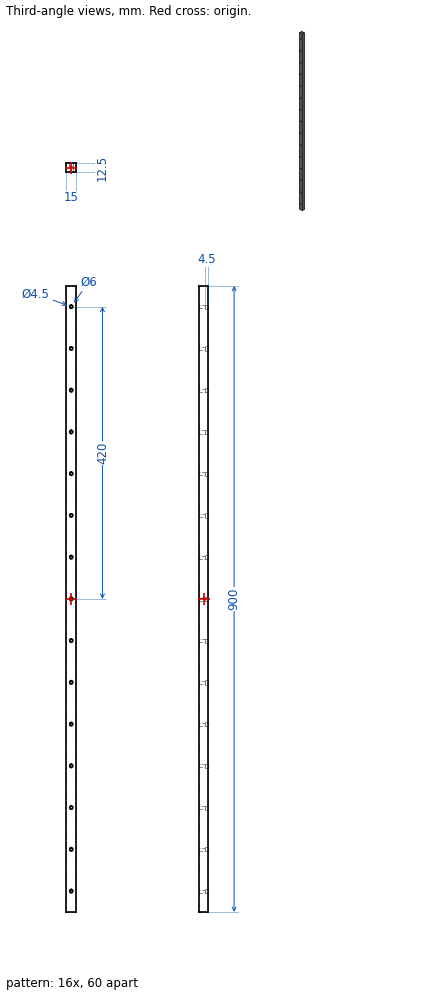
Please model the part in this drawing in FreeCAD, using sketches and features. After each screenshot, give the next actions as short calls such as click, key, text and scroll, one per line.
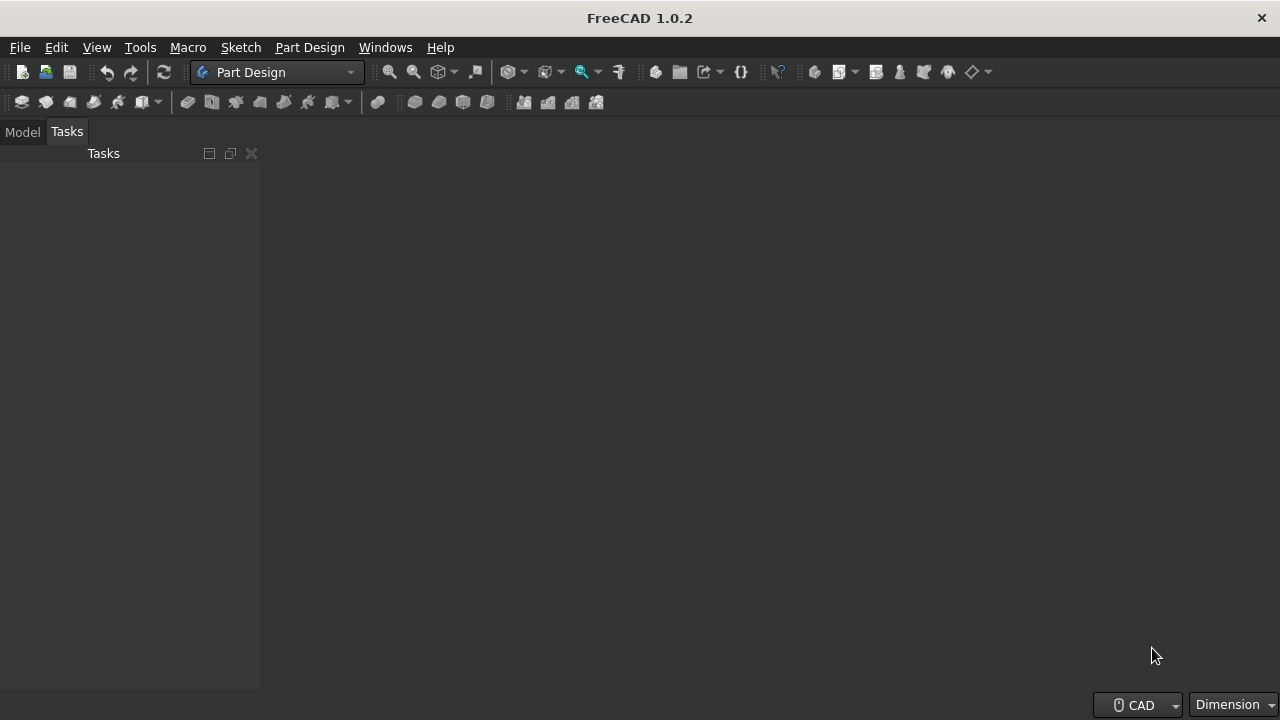
click(22, 72)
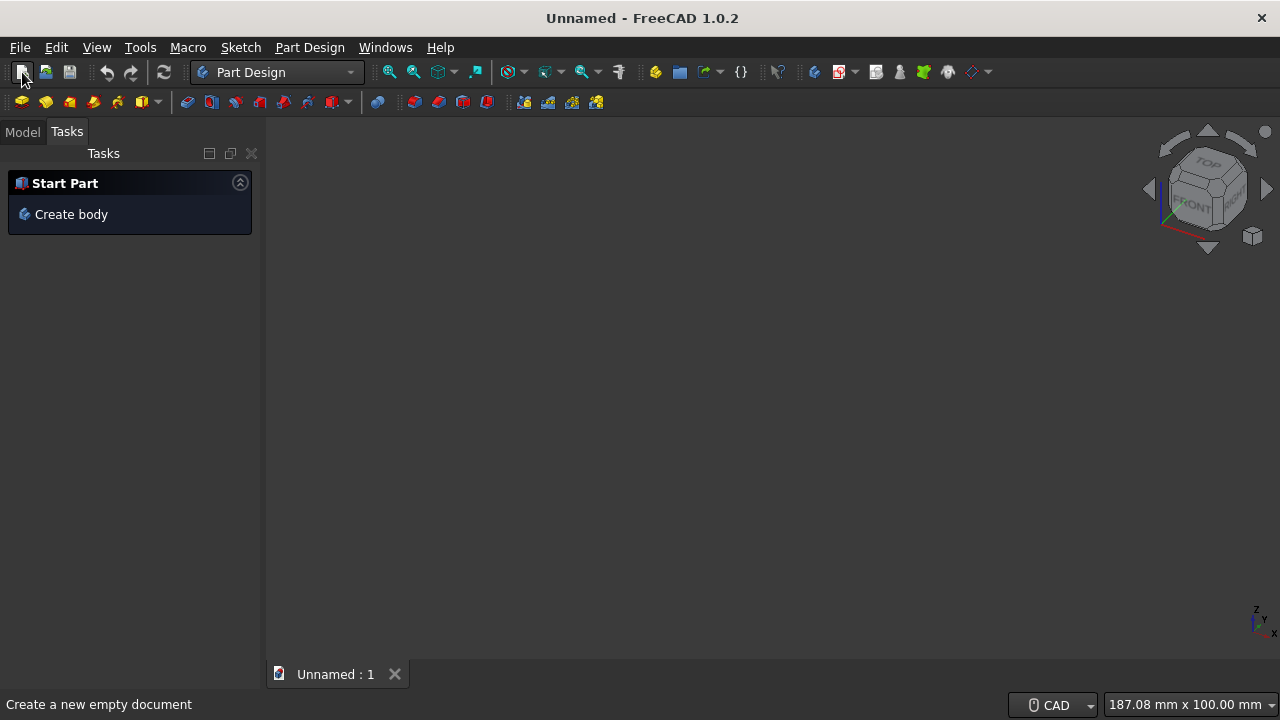
click(840, 72)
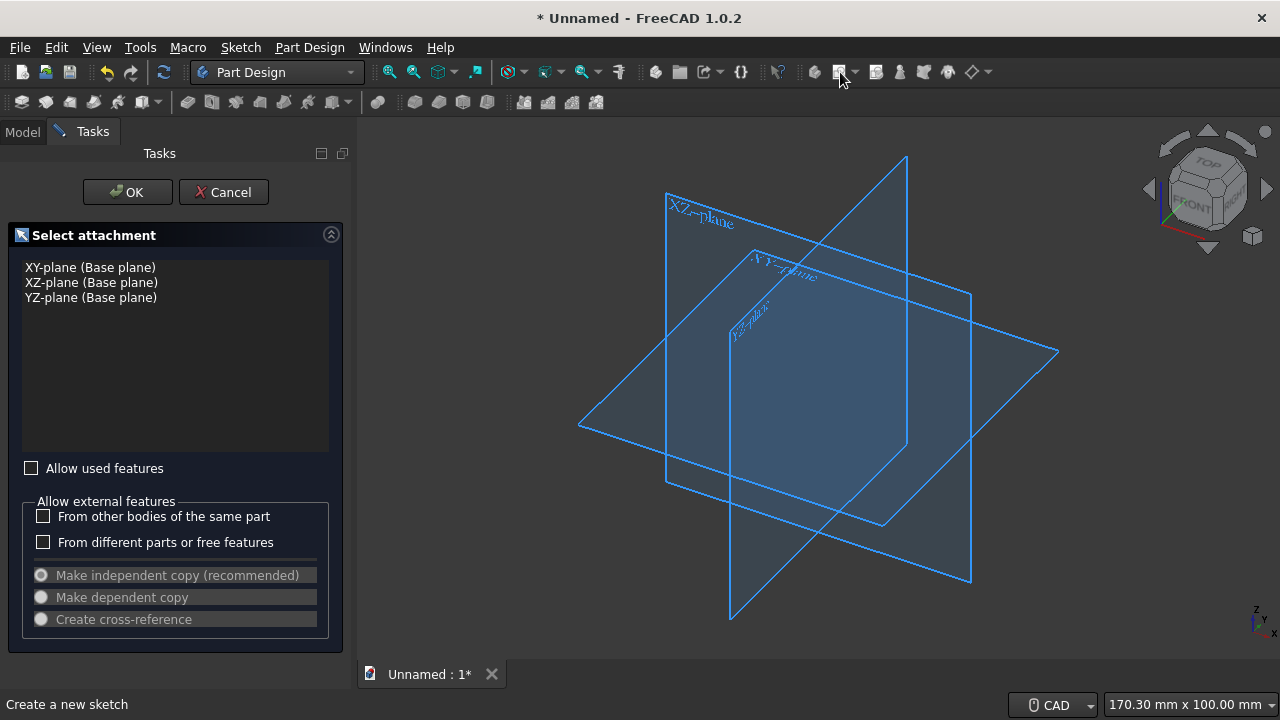
click(82, 268)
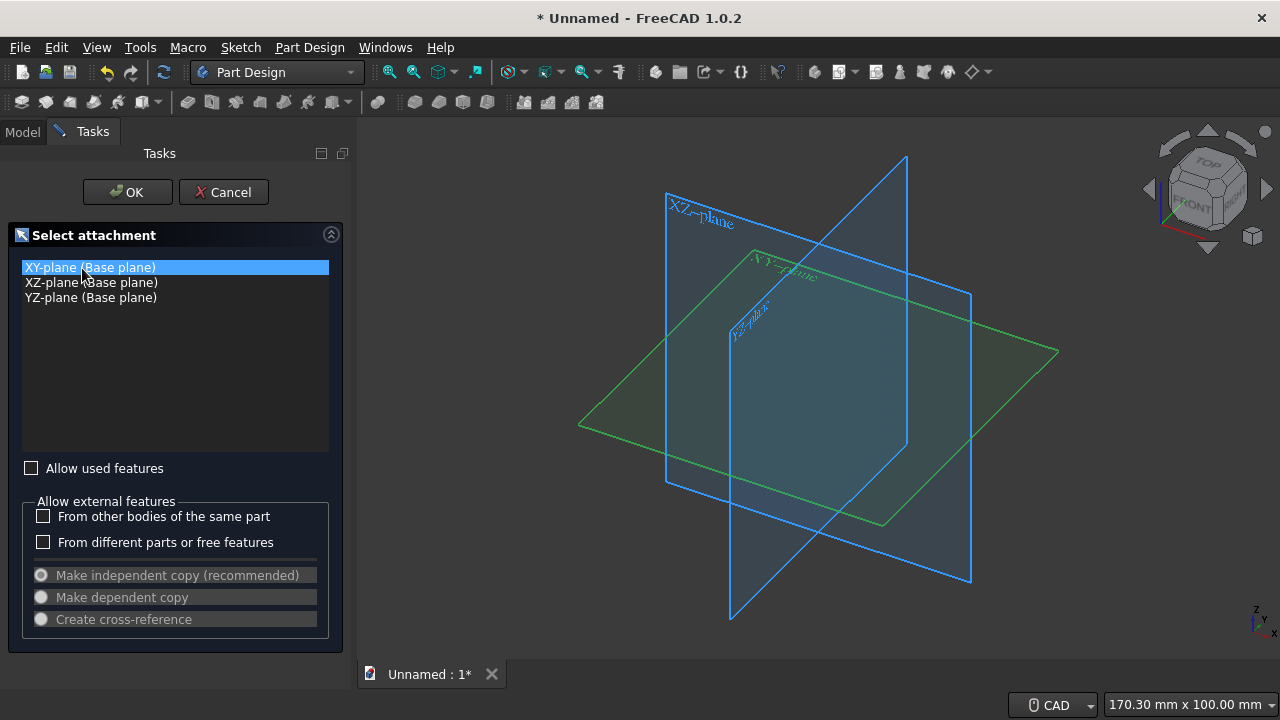
click(128, 192)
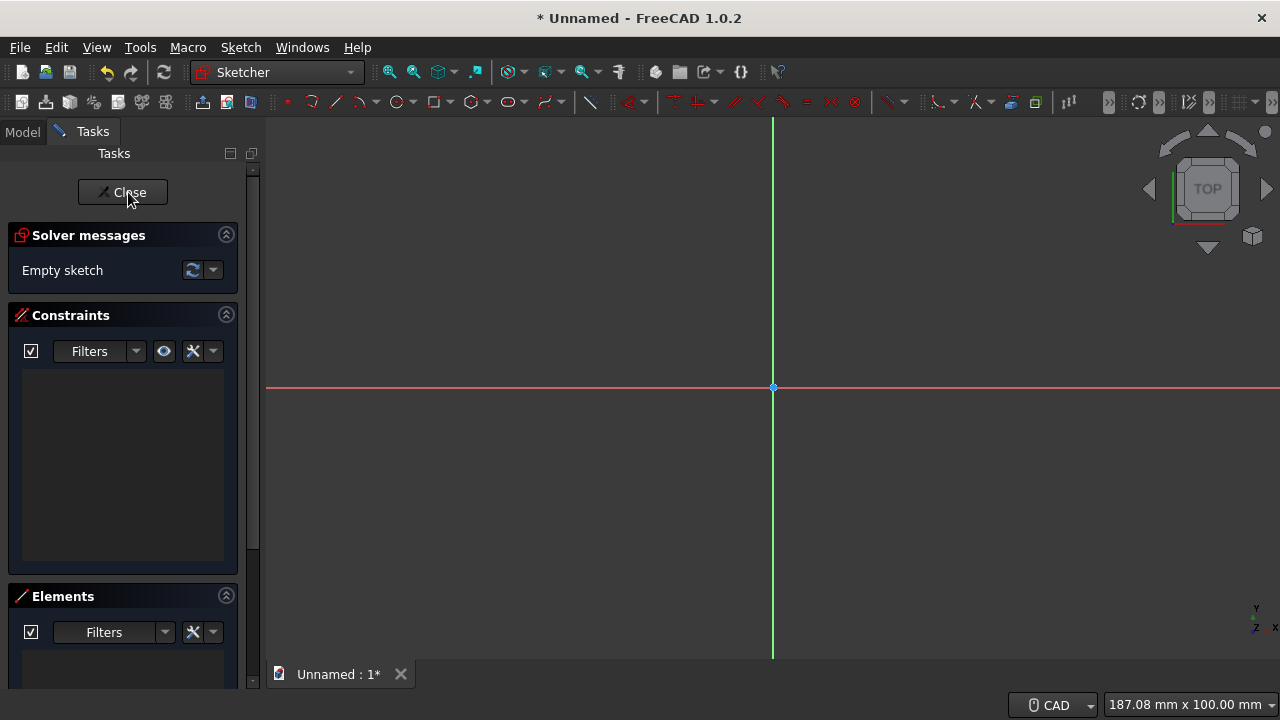
scroll(790, 388, up, 8)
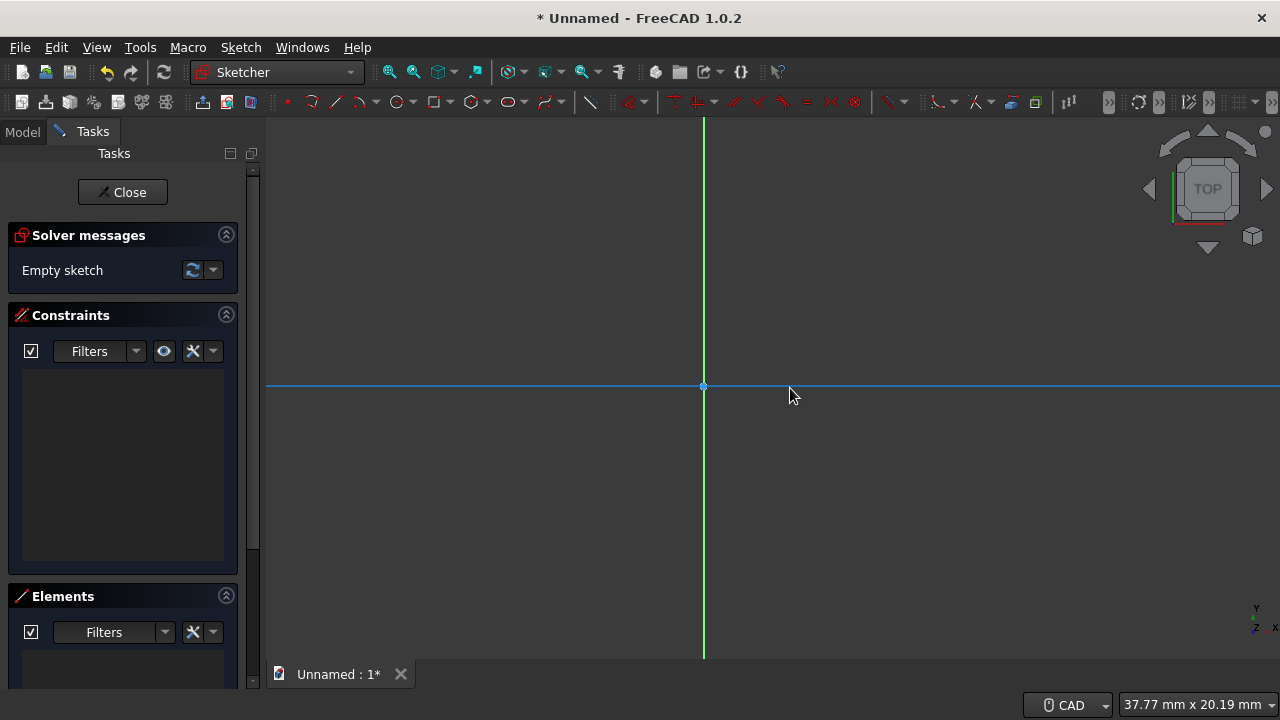
key(g)
key(v)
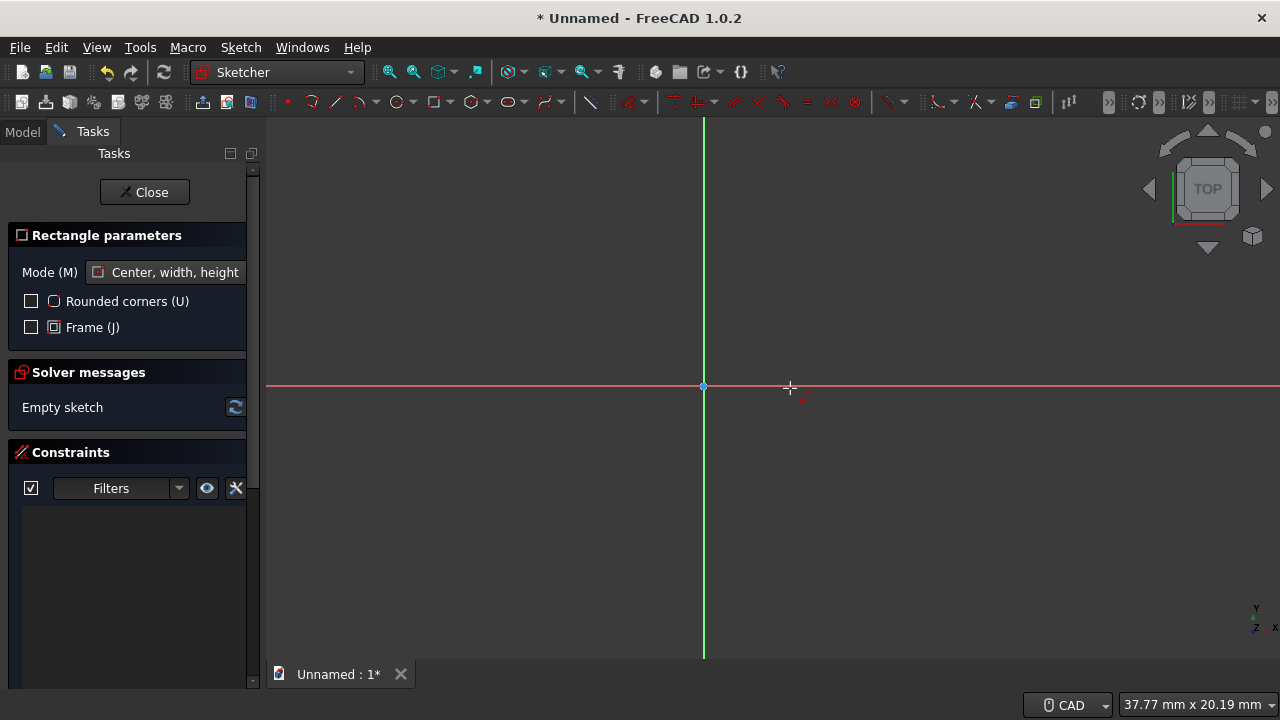
click(704, 386)
move(905, 218)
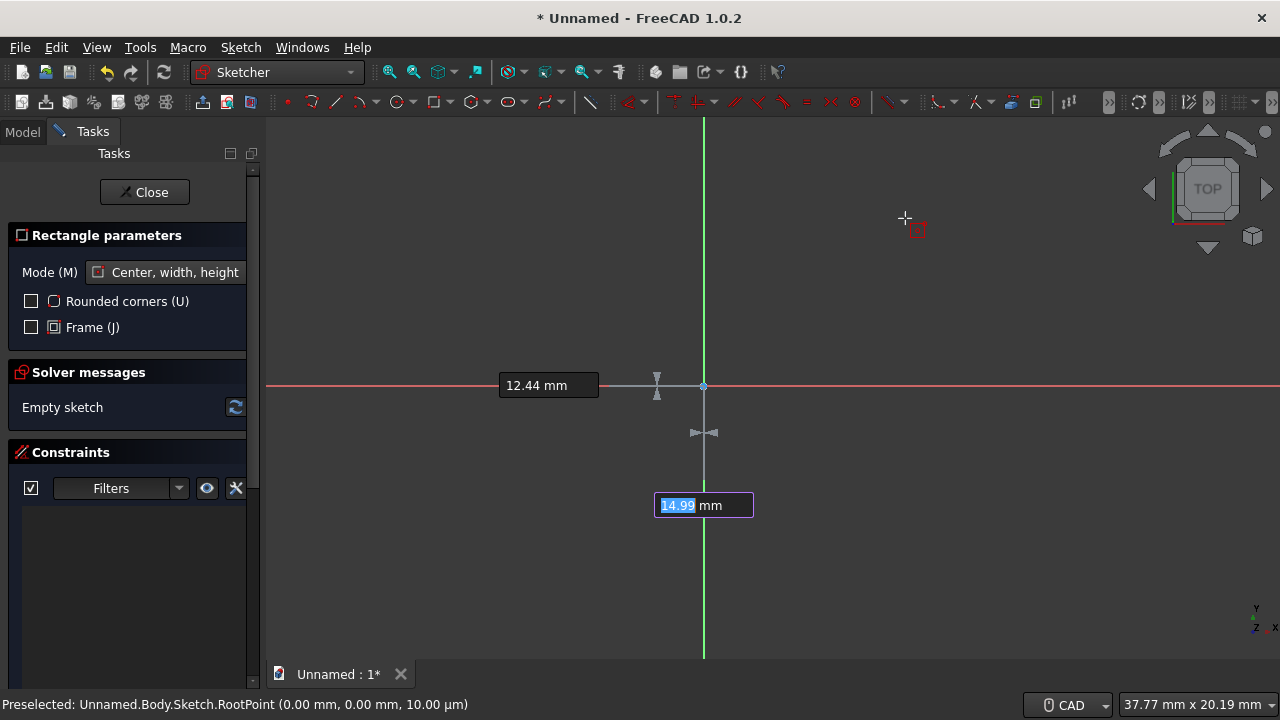
text(15)
key(Tab)
text(12.5)
key(Return)
key(Escape)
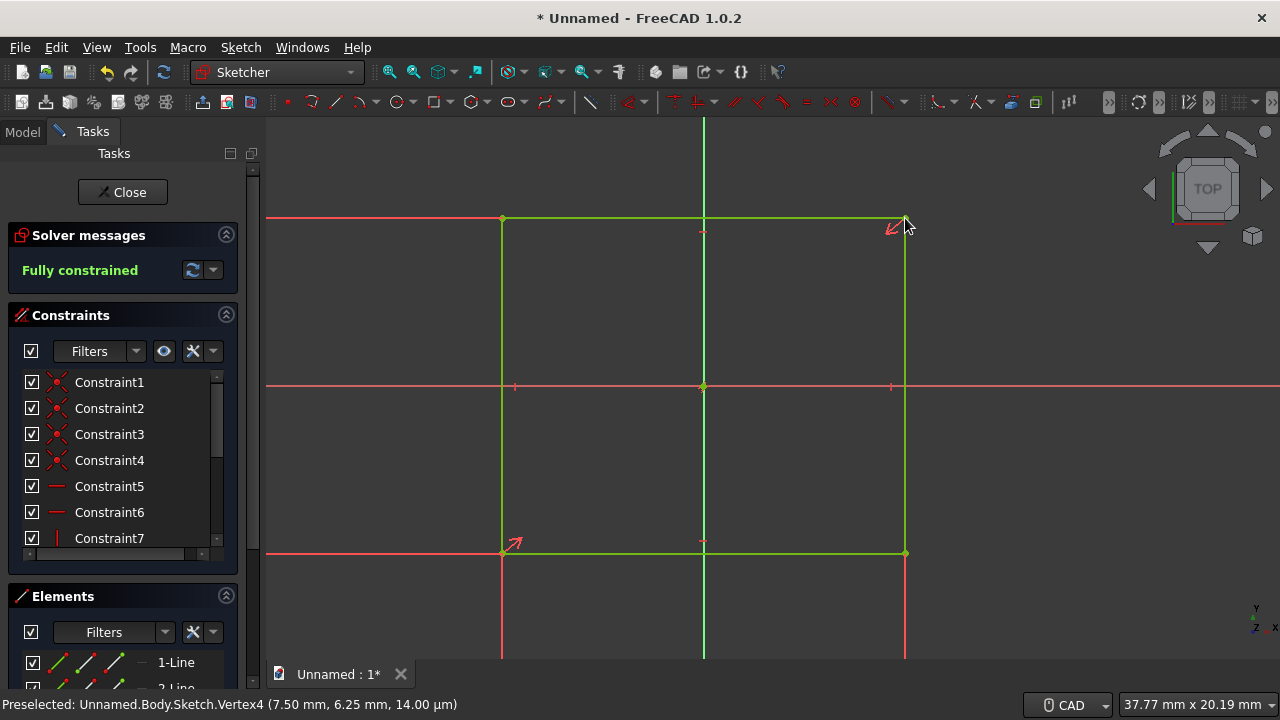
click(123, 192)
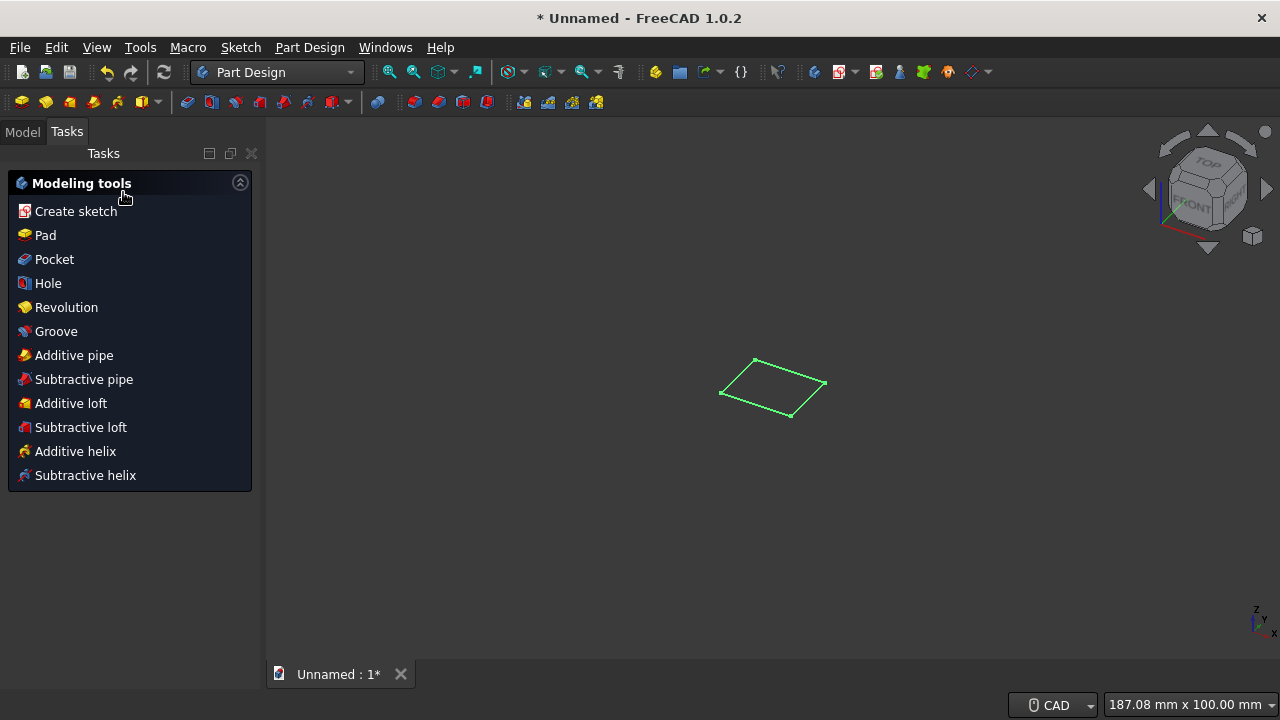
click(22, 102)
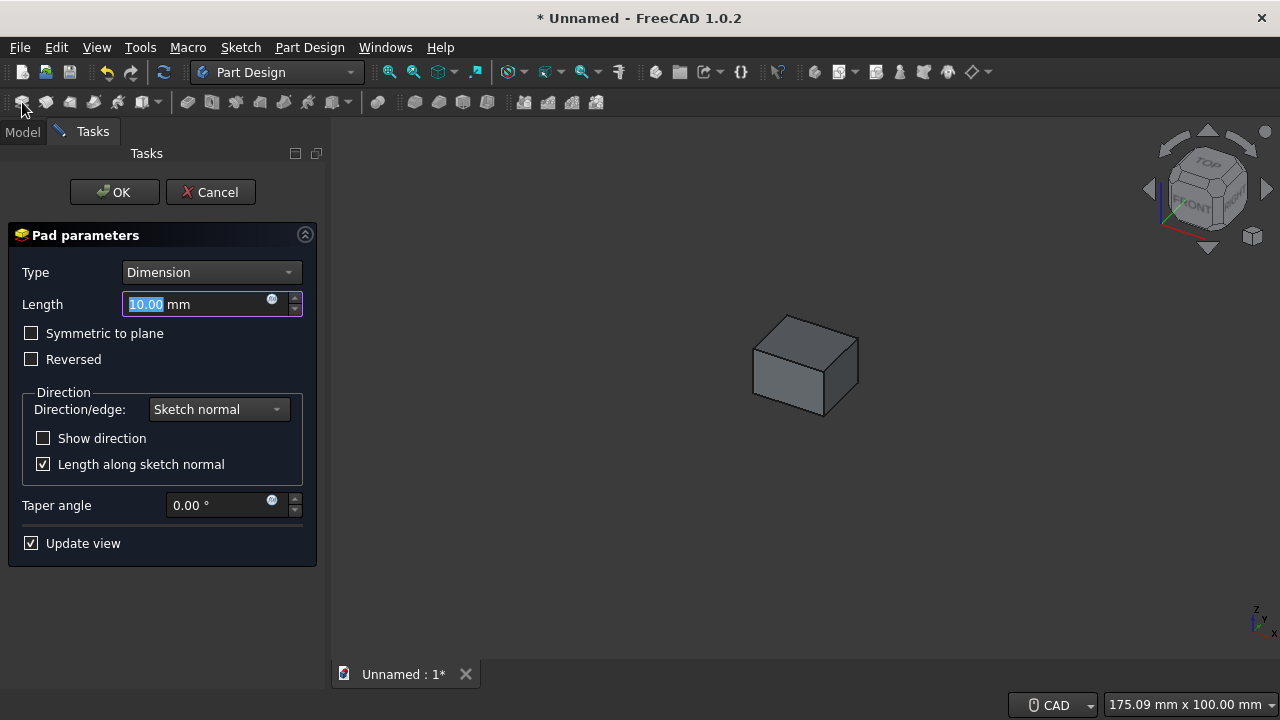
text(900)
key(Tab)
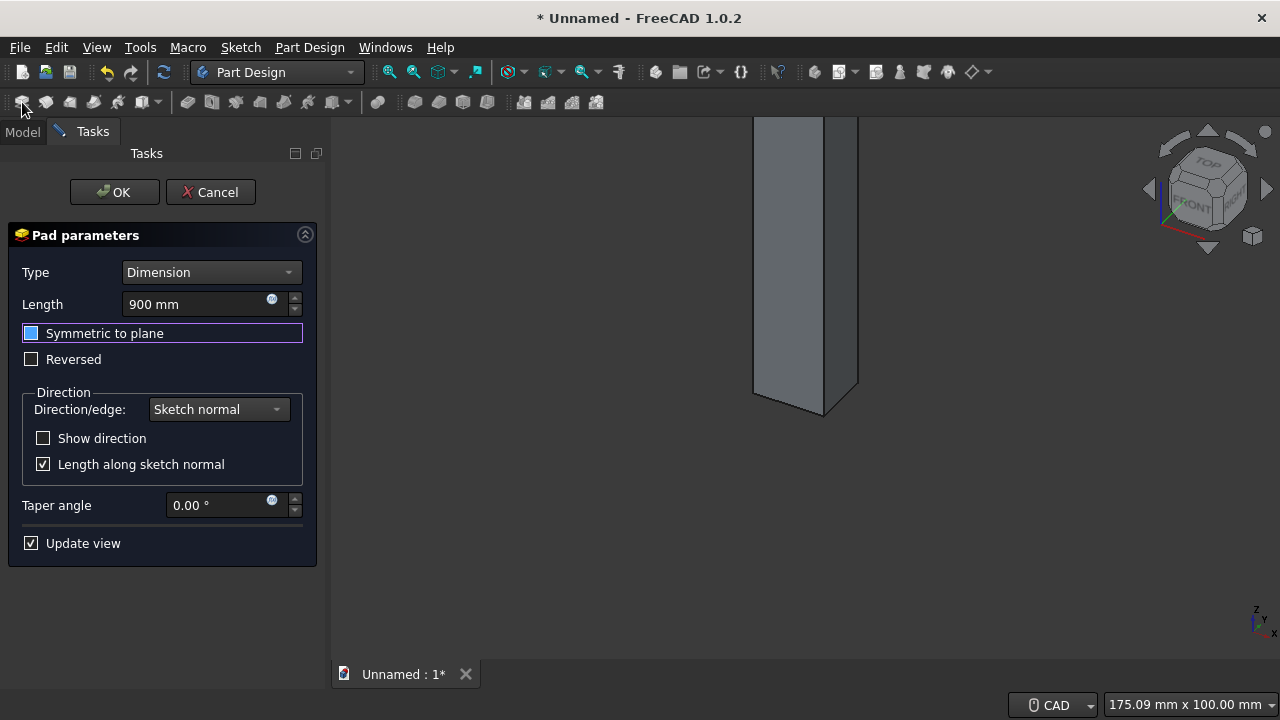
click(30, 333)